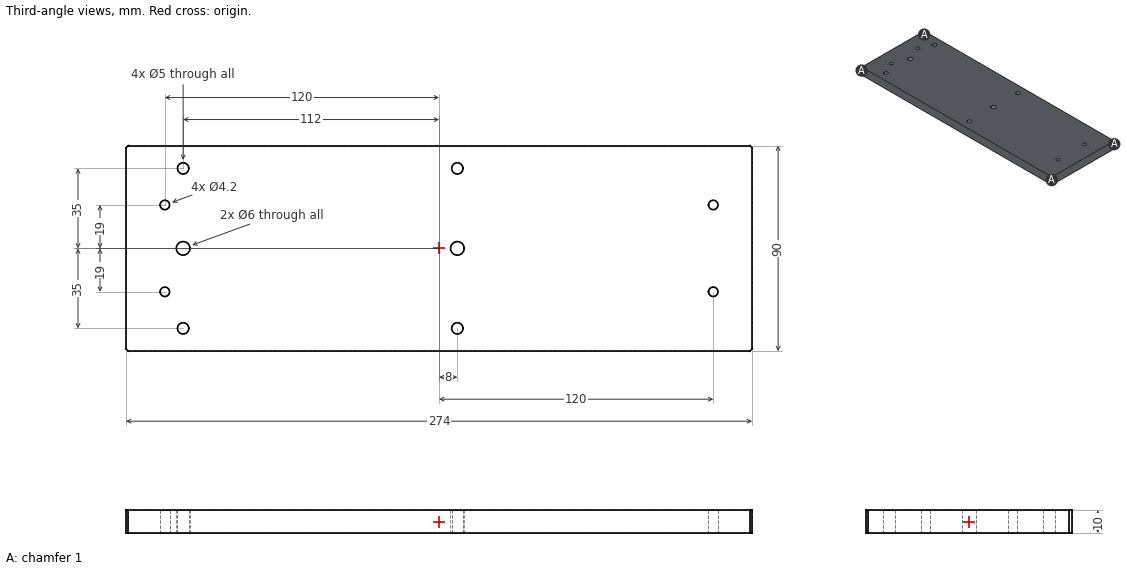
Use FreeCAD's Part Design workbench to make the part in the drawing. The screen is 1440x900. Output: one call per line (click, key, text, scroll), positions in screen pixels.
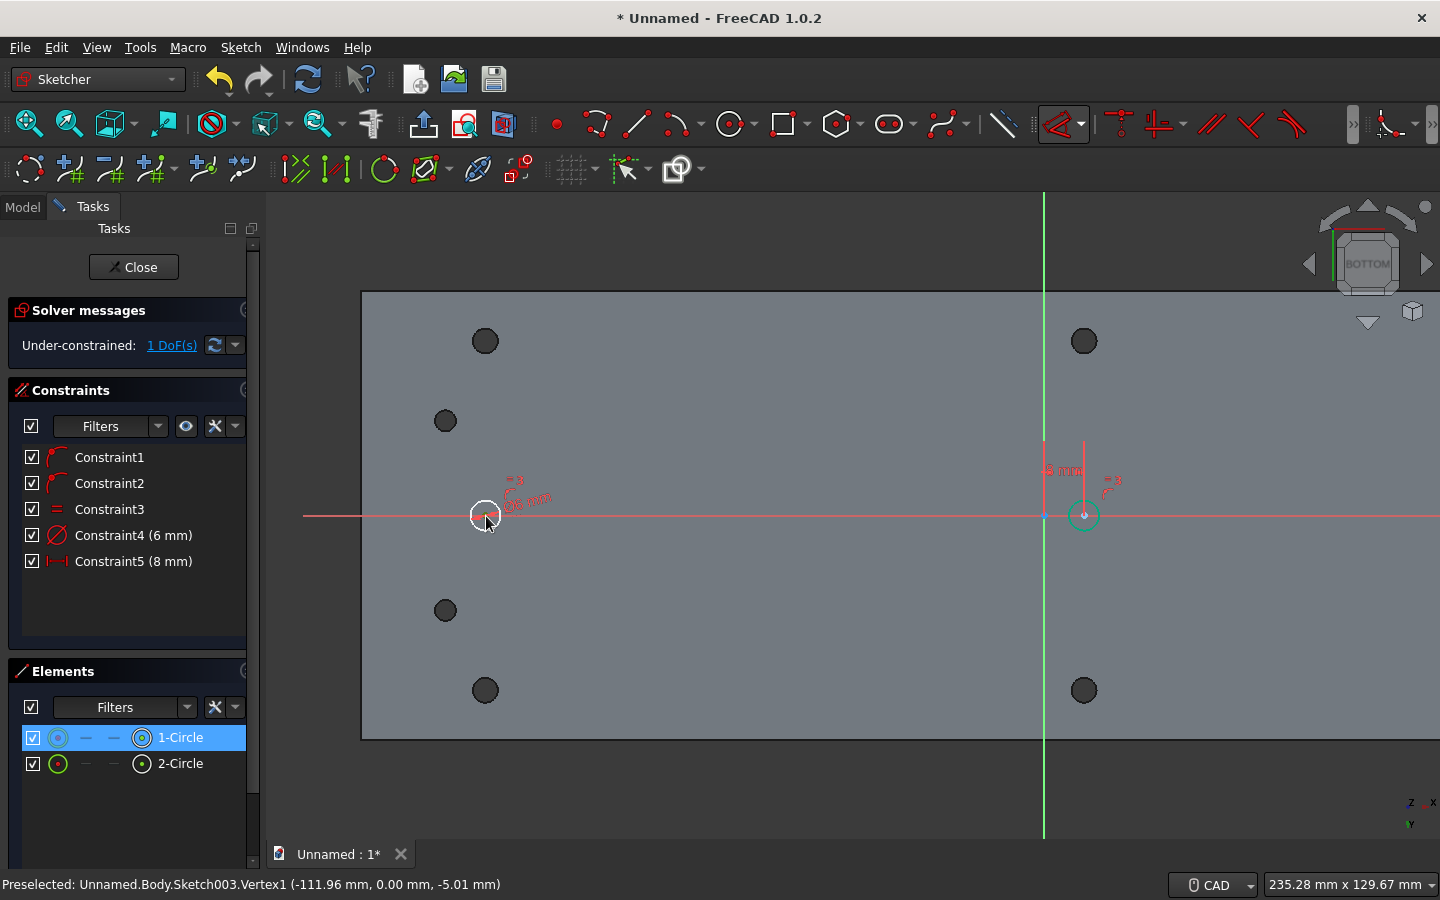
key(l)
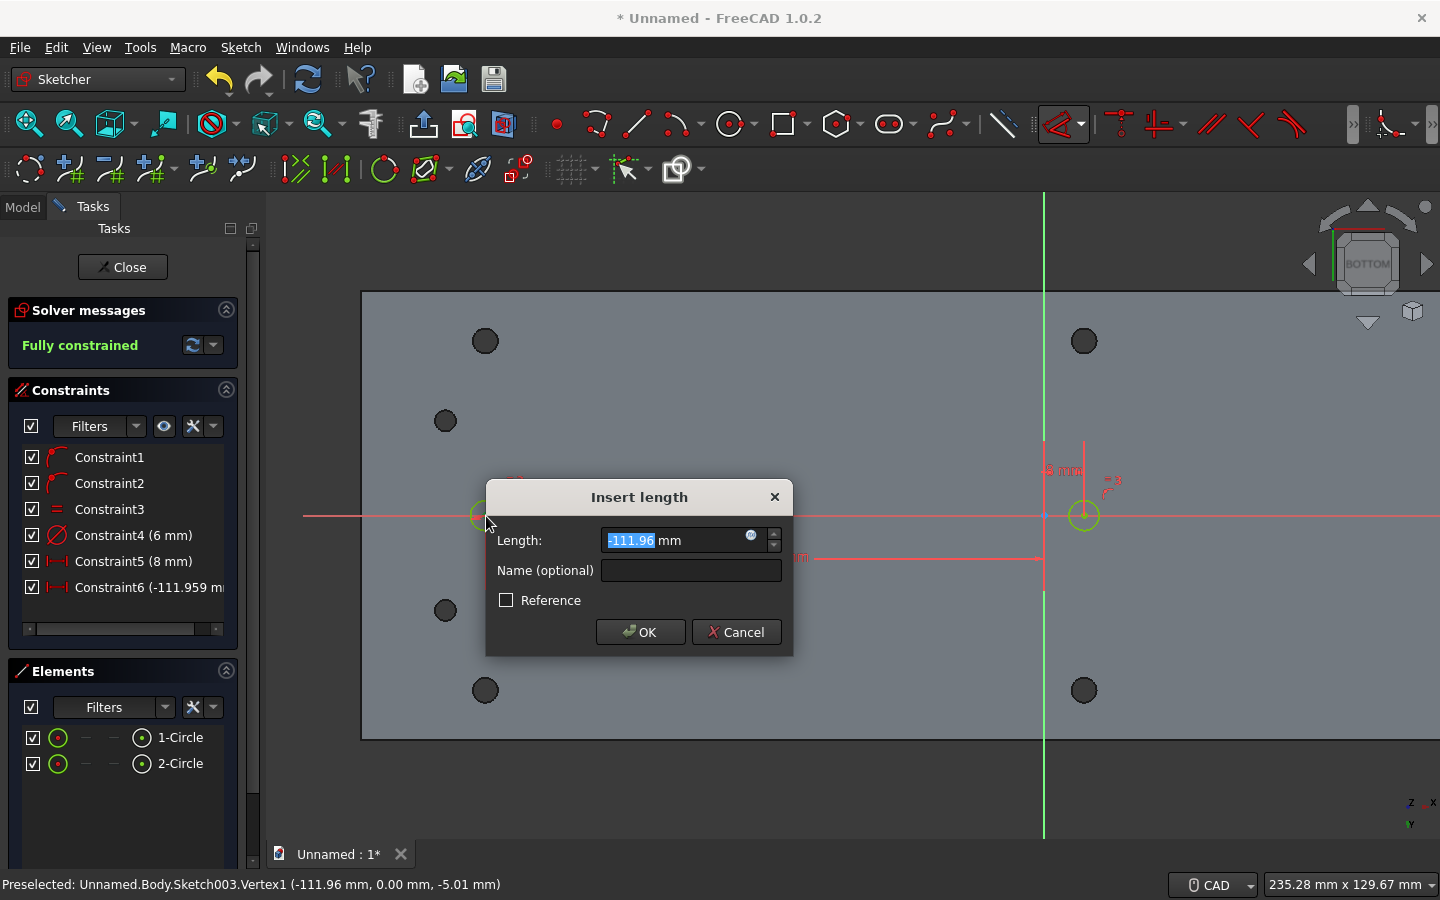
text(-112)
key(Return)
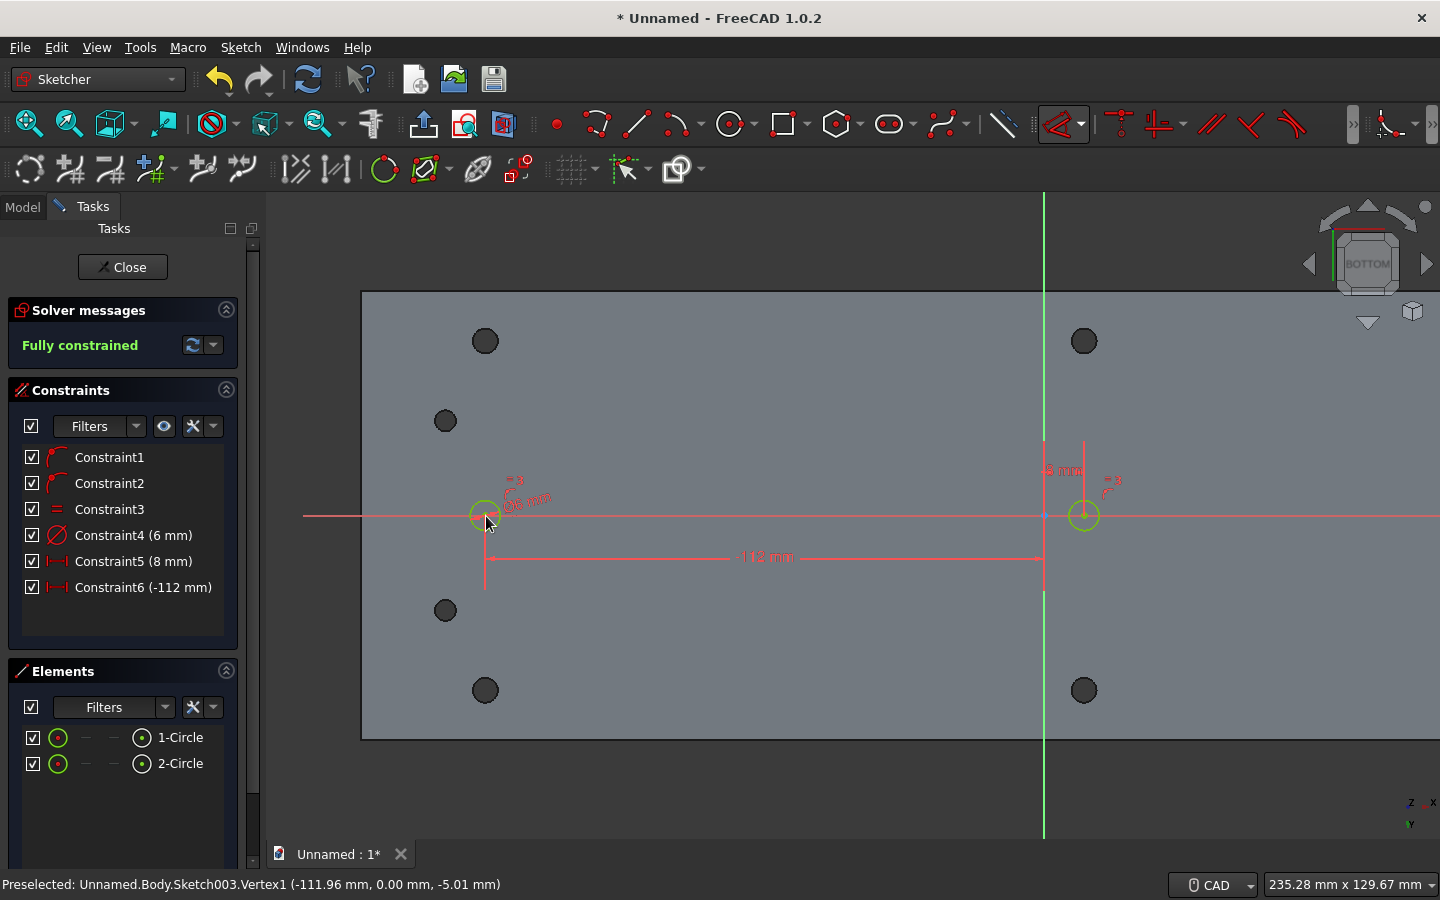
click(123, 267)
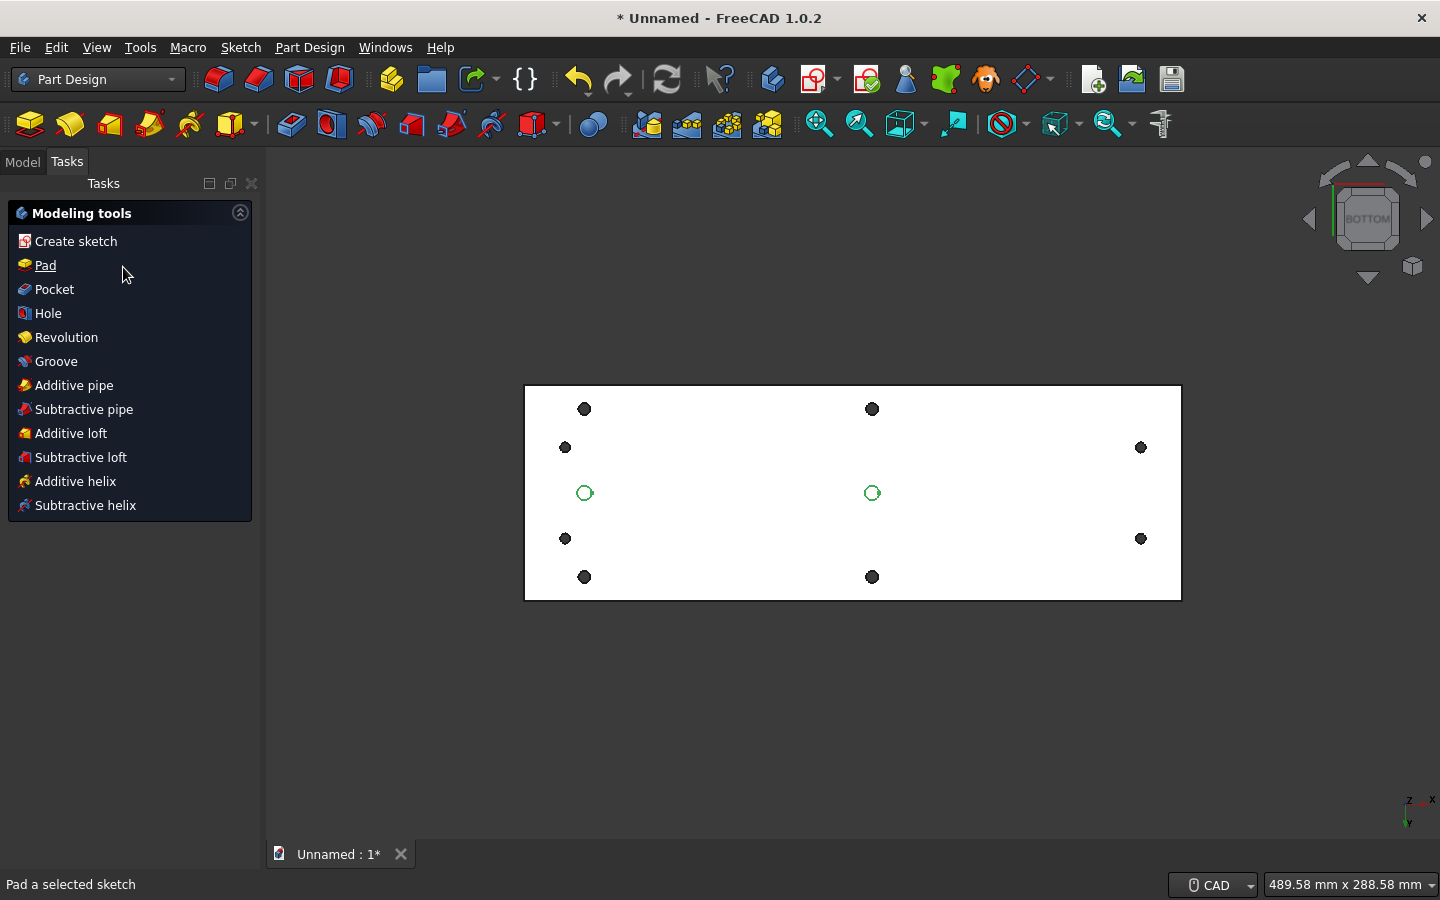
click(332, 124)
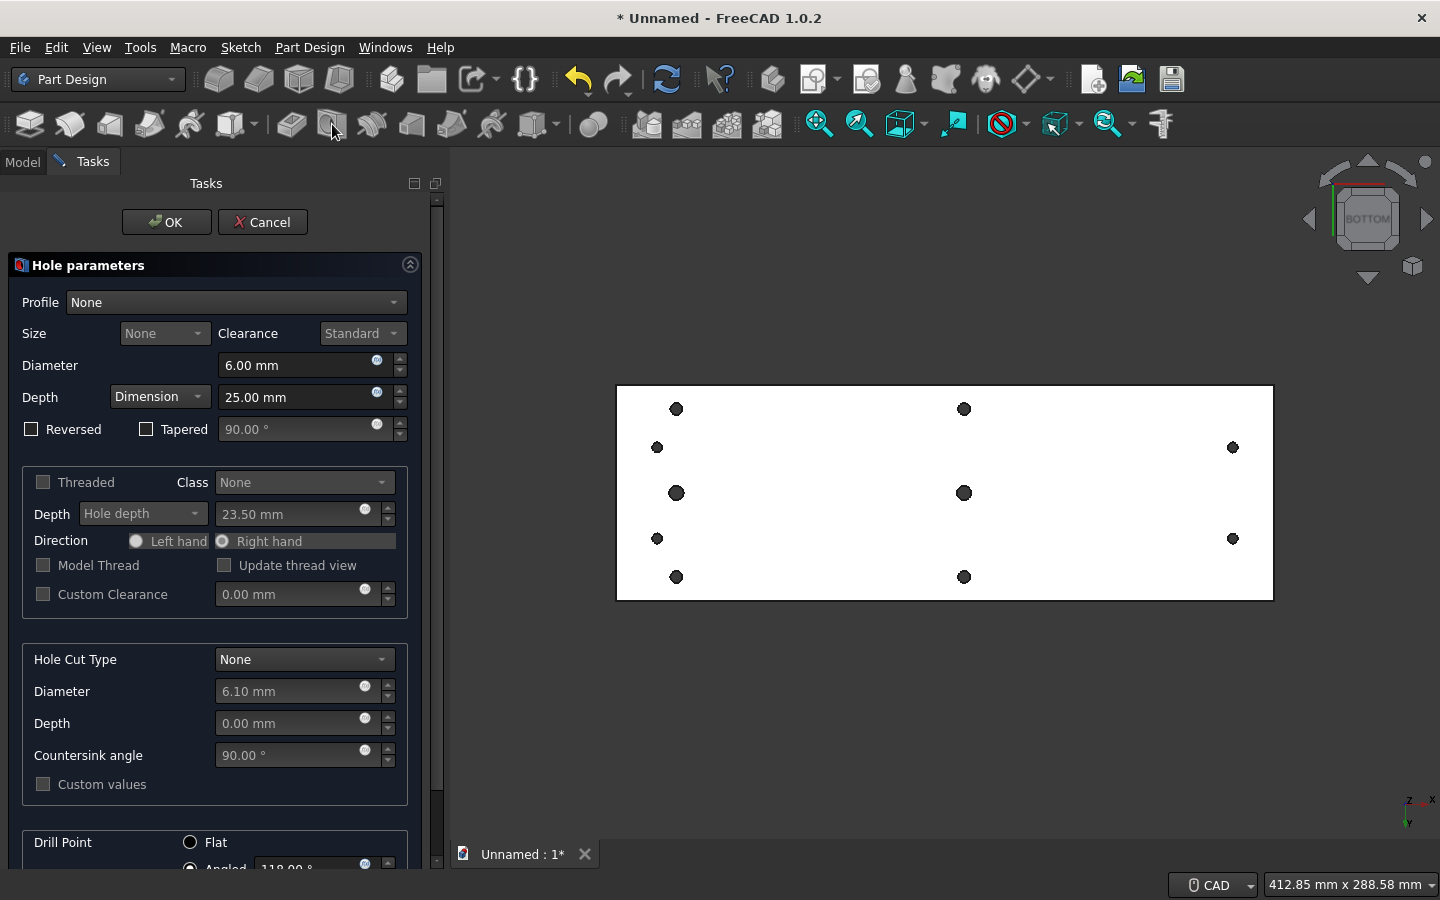
triple_click(305, 365)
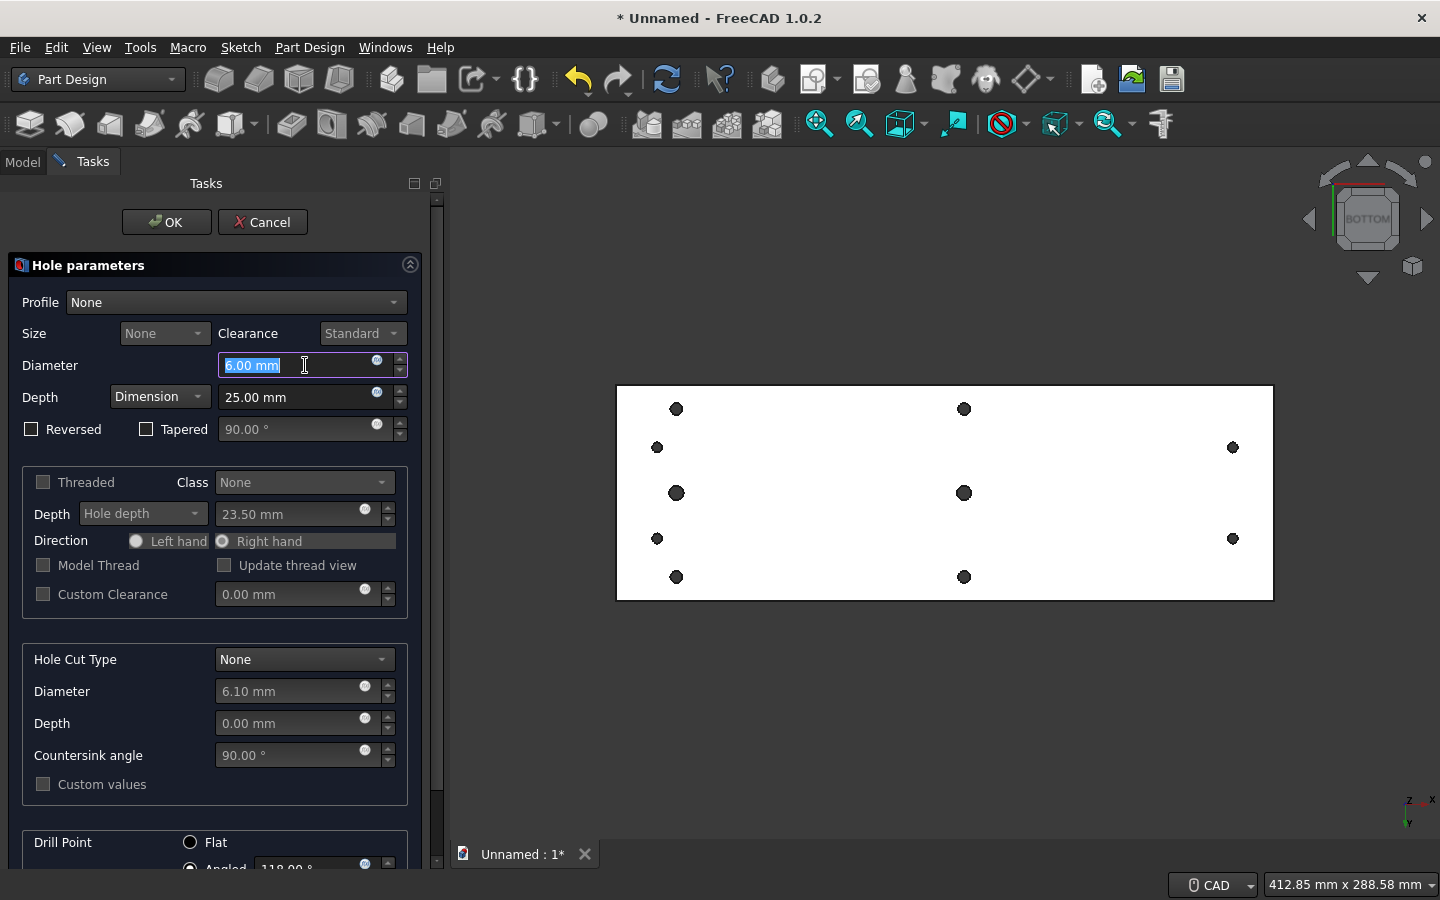
text(6)
key(Tab)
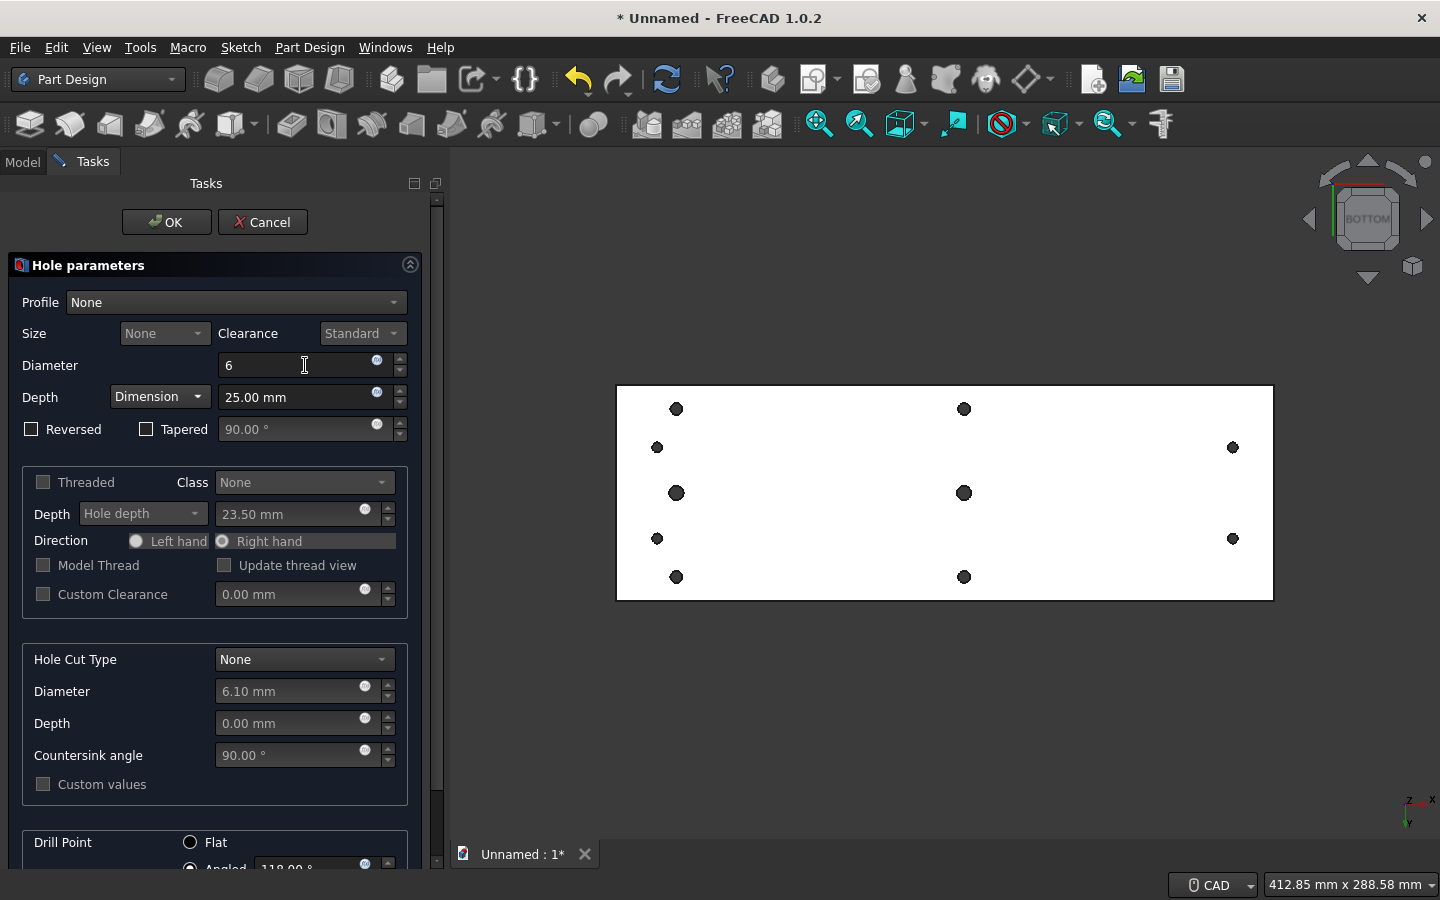
click(161, 396)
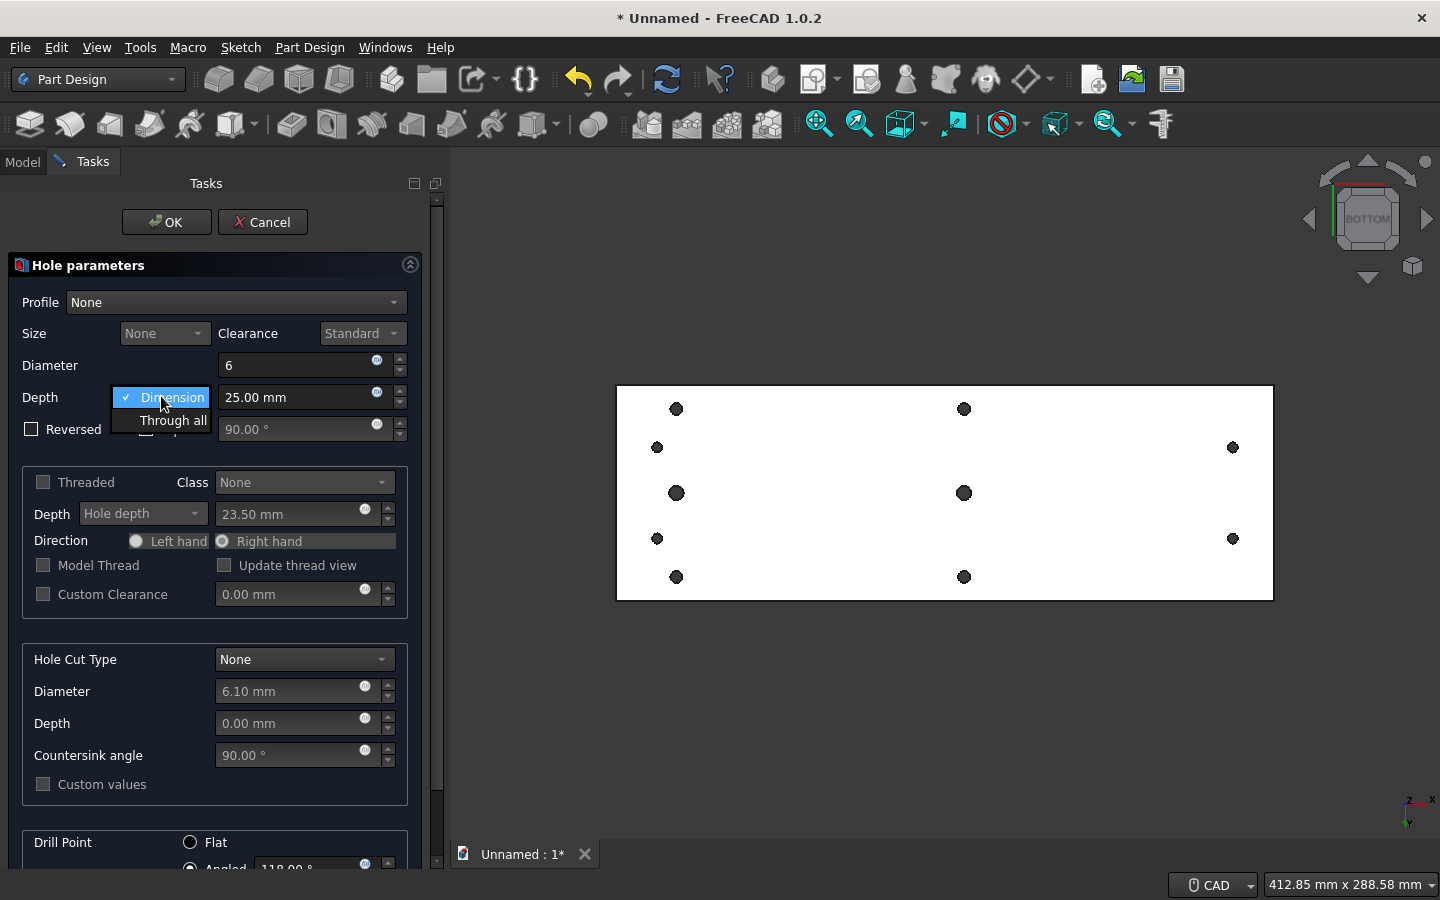
click(160, 420)